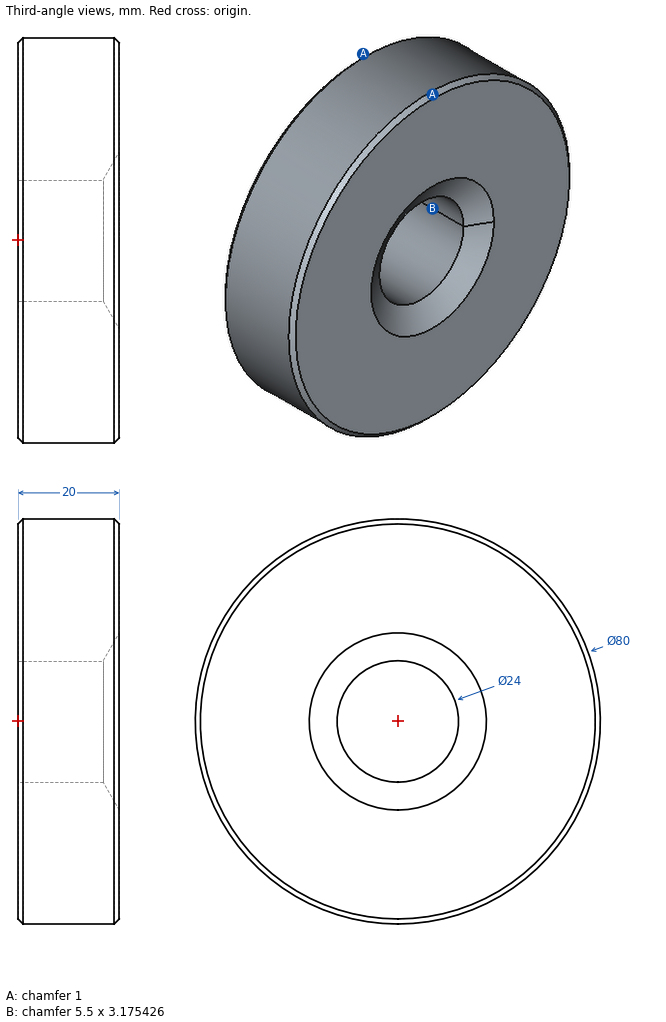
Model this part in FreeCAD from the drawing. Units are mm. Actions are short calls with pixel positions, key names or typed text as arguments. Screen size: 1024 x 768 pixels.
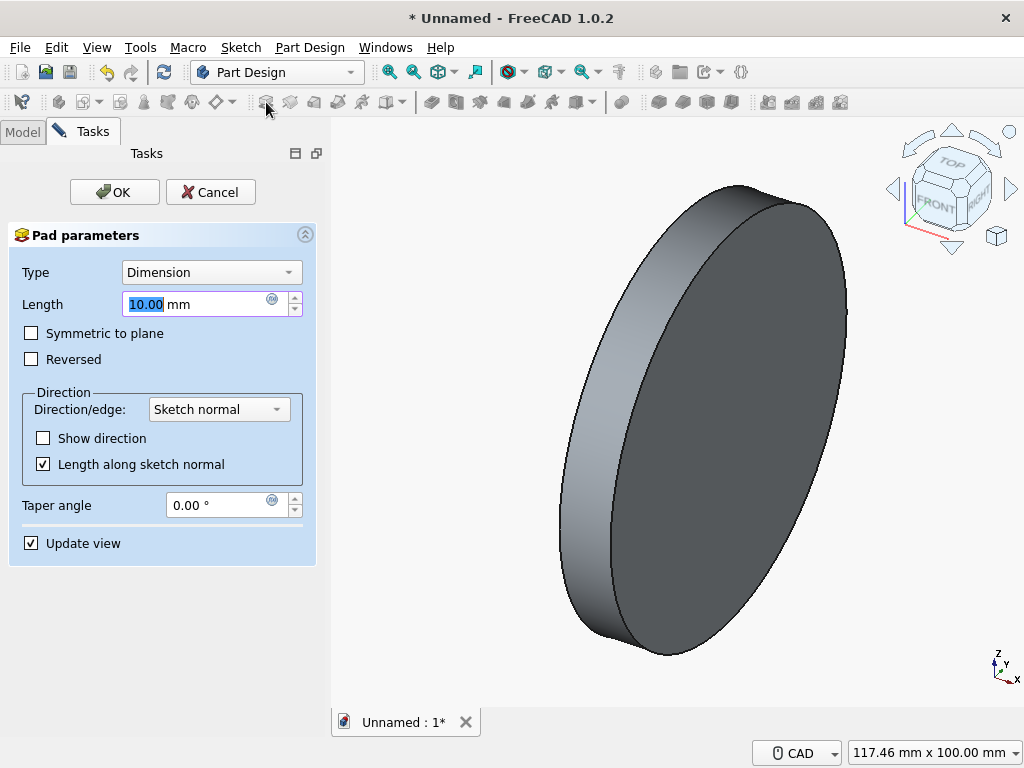
text(20)
key(Tab)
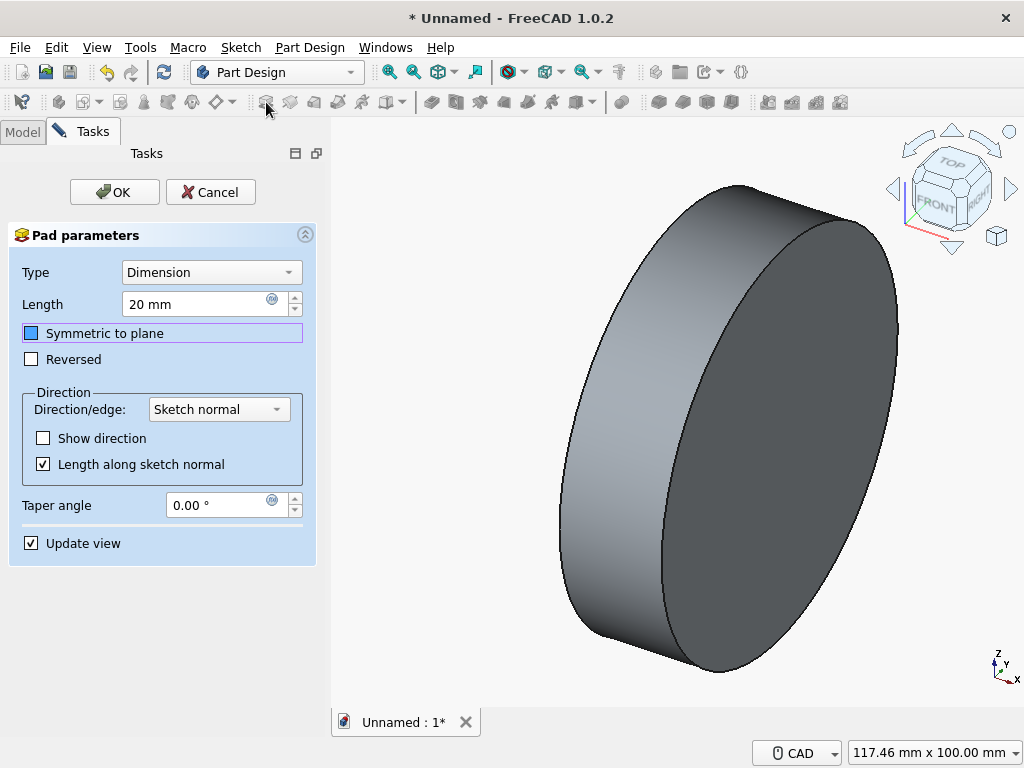
click(115, 192)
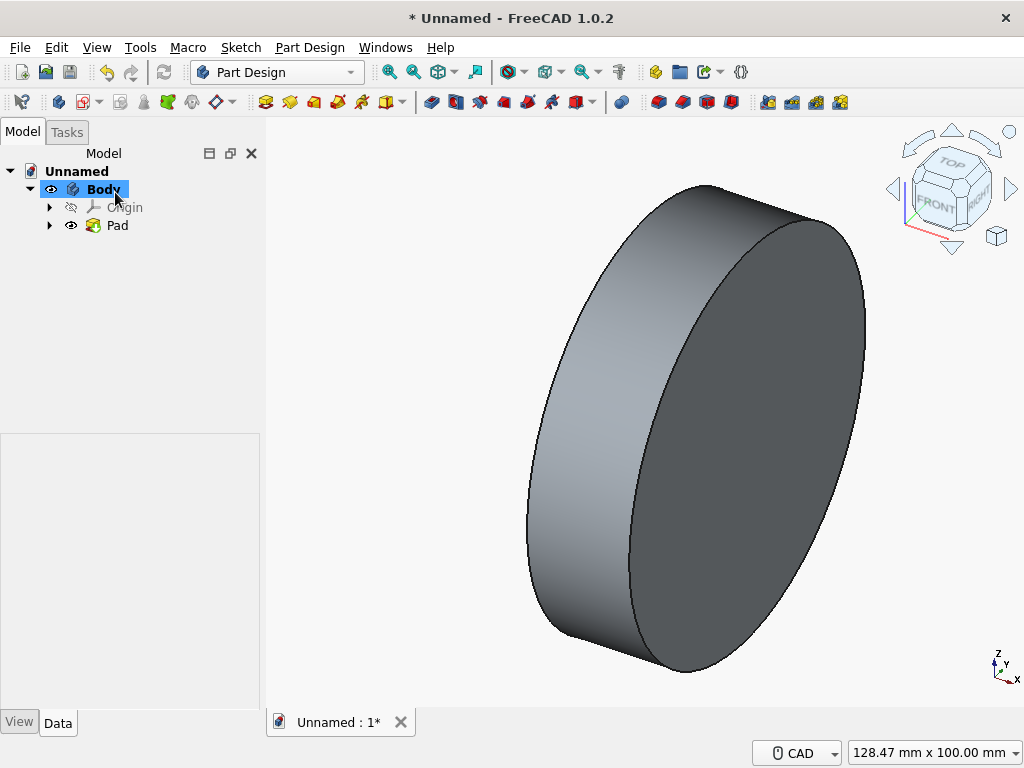
click(390, 72)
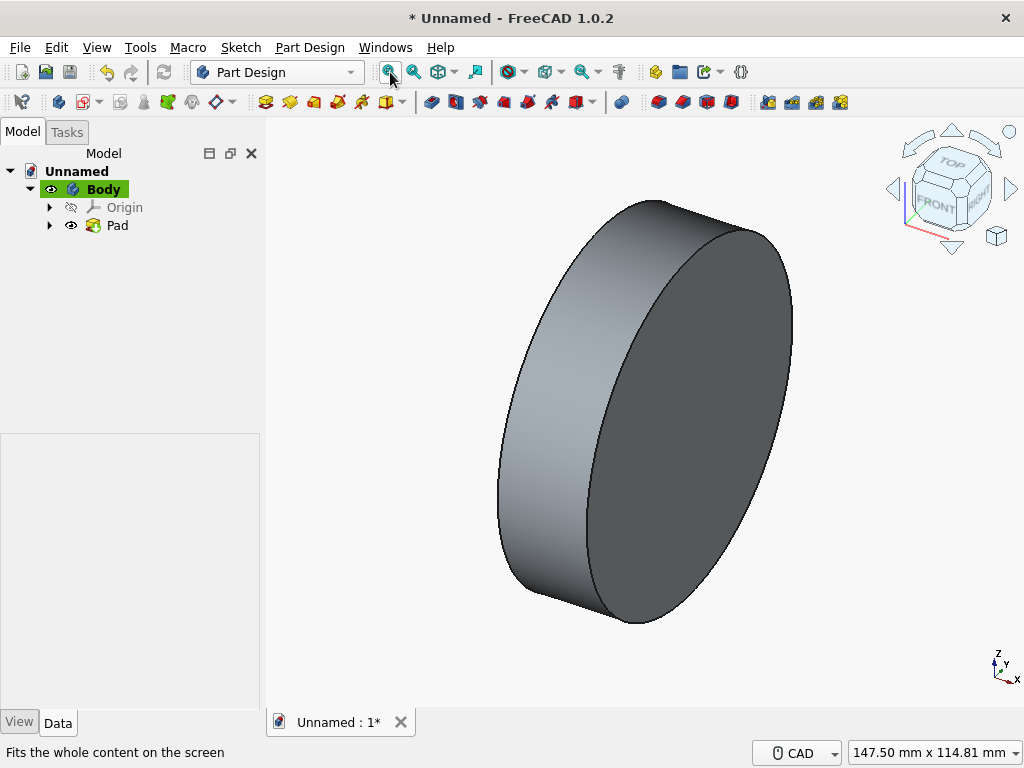
click(690, 426)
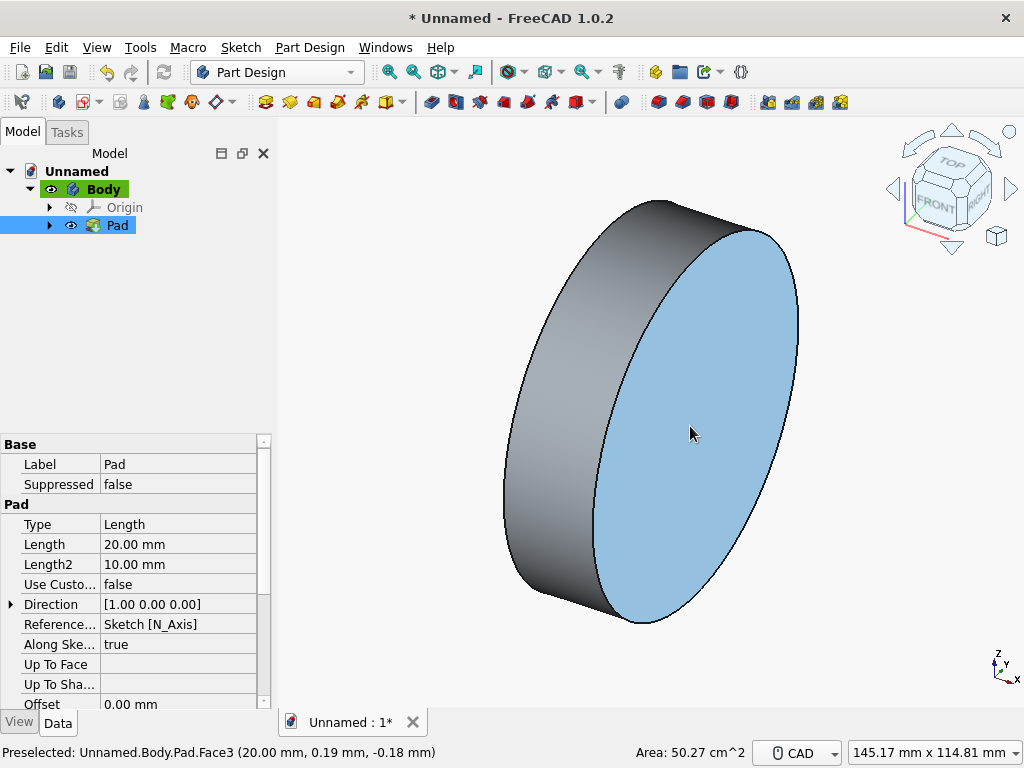
click(84, 102)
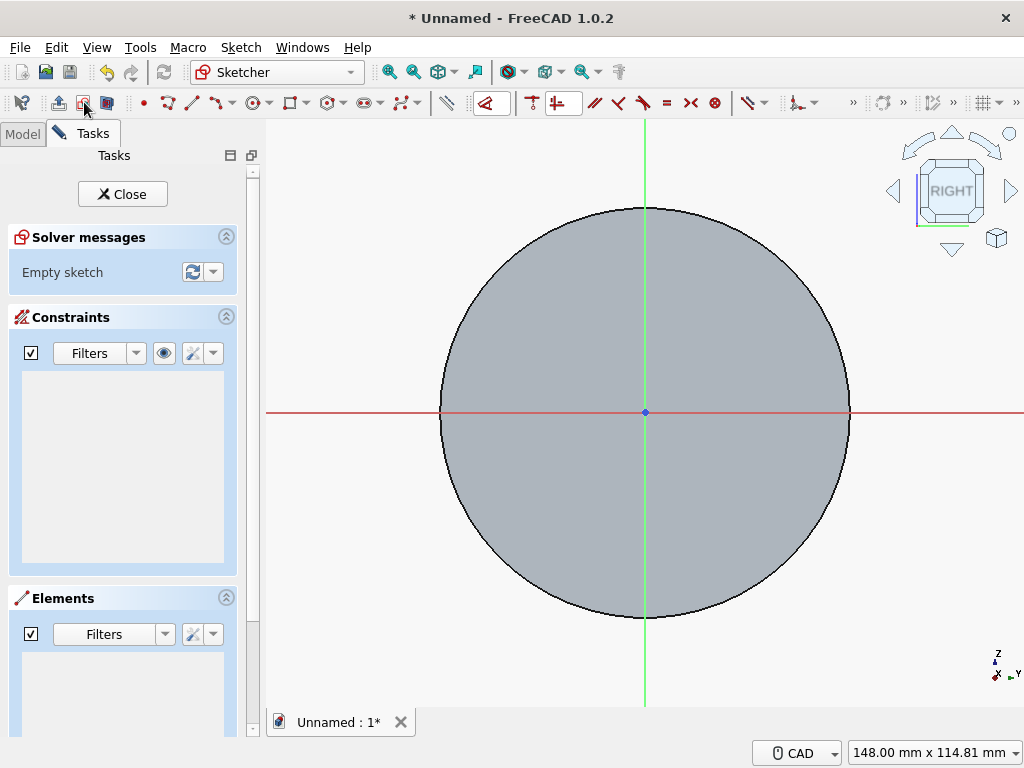
scroll(675, 413, up, 6)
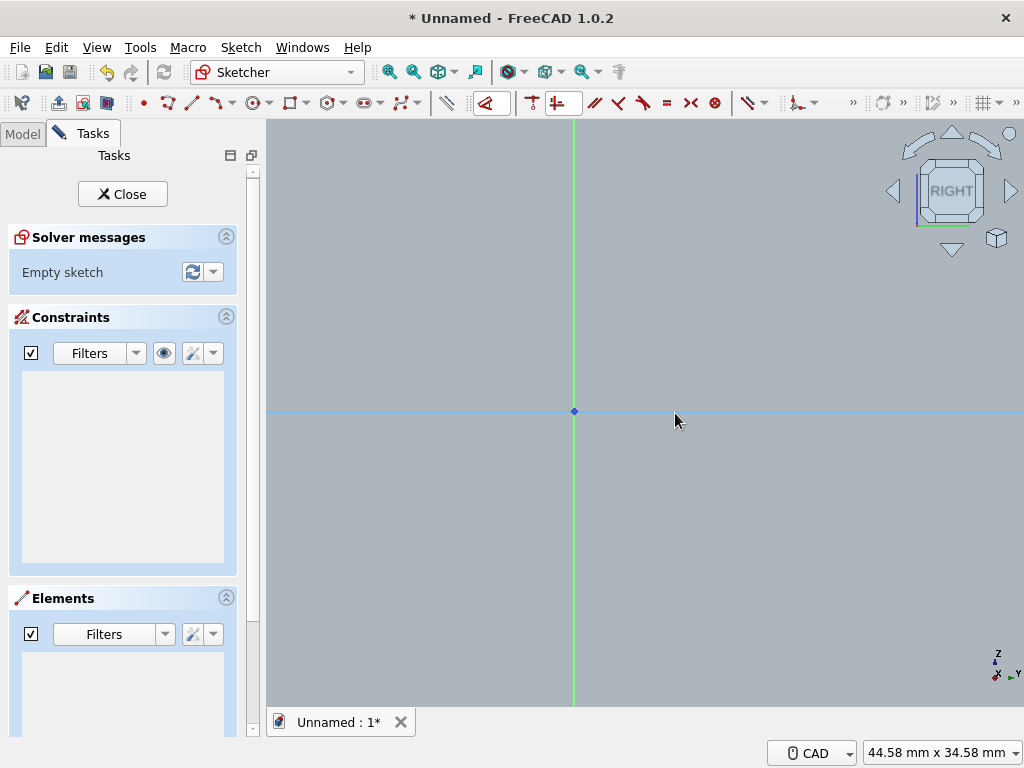
click(254, 104)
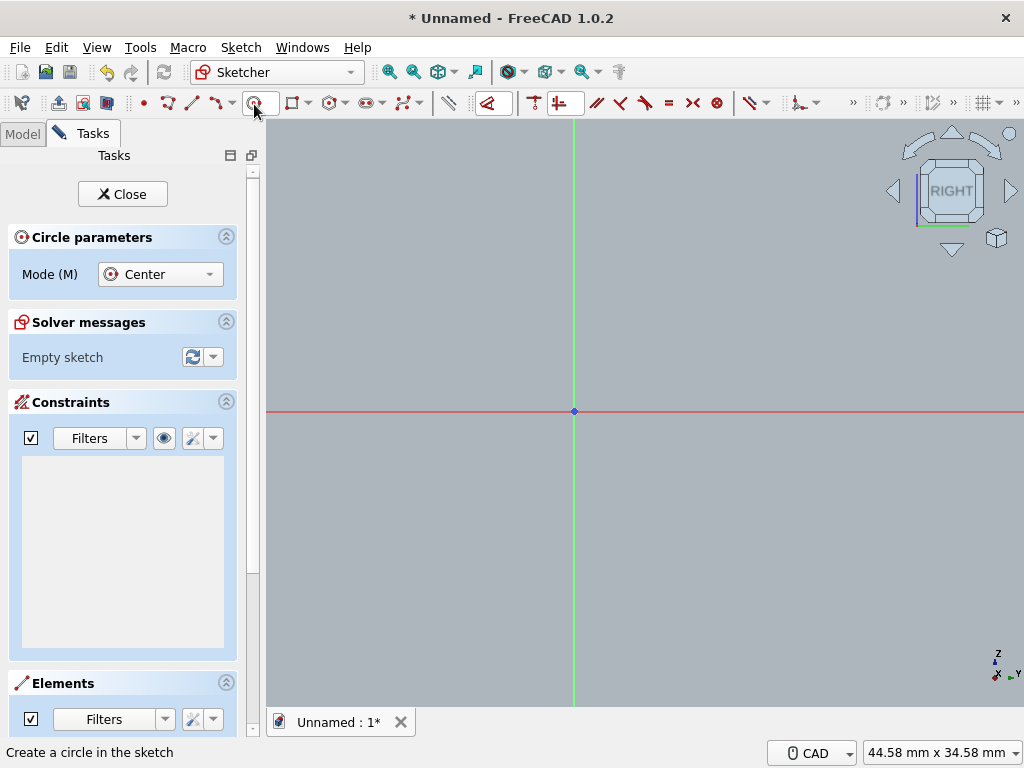
click(574, 412)
click(718, 268)
key(Escape)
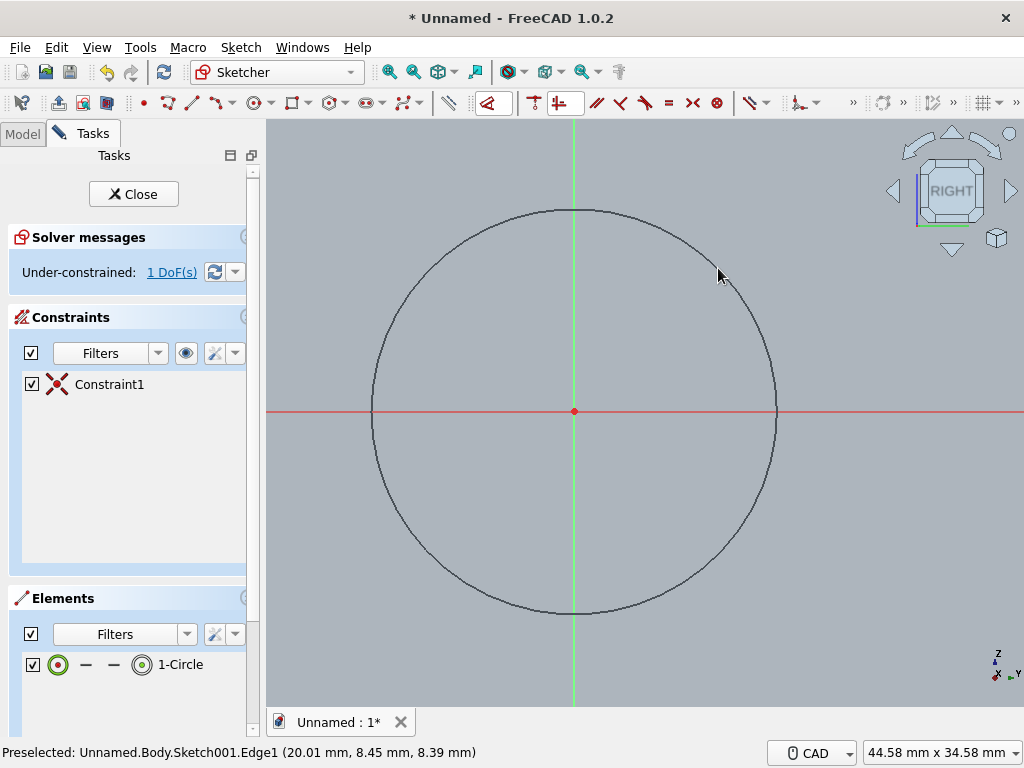
click(717, 268)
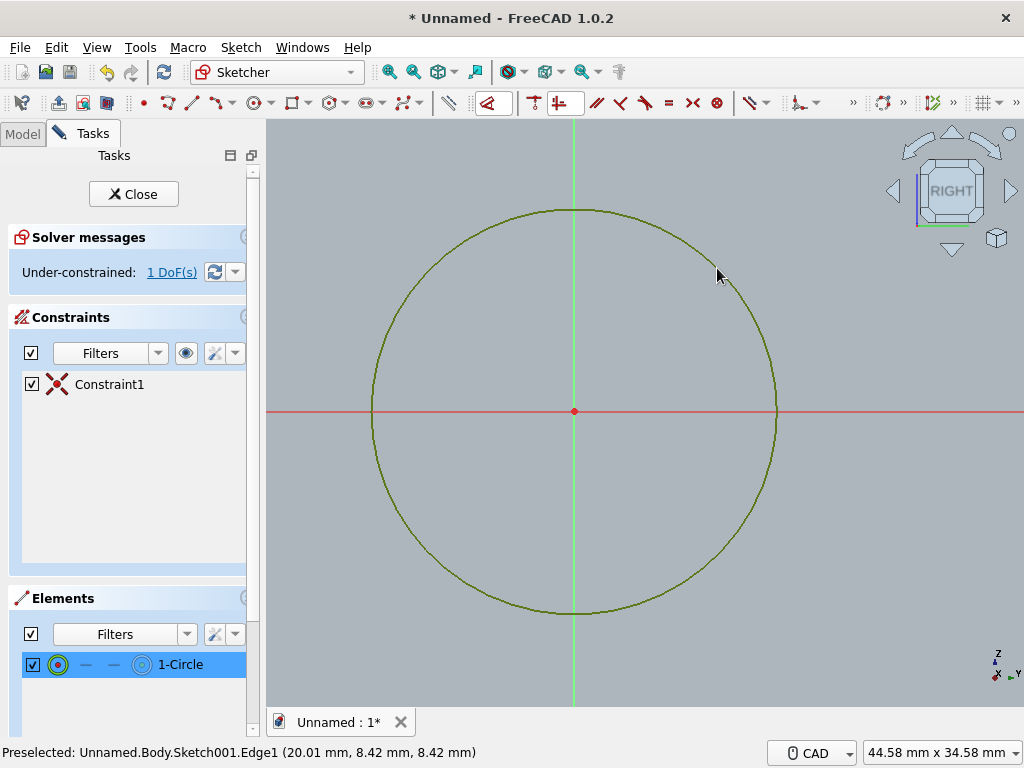
click(506, 104)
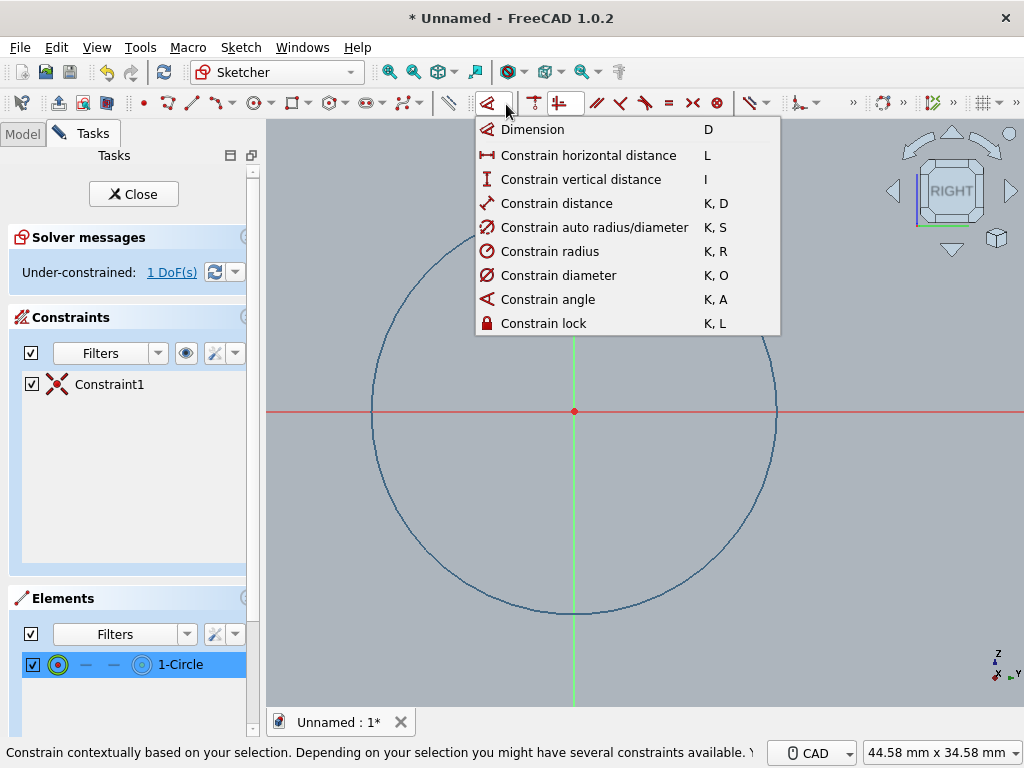
click(628, 275)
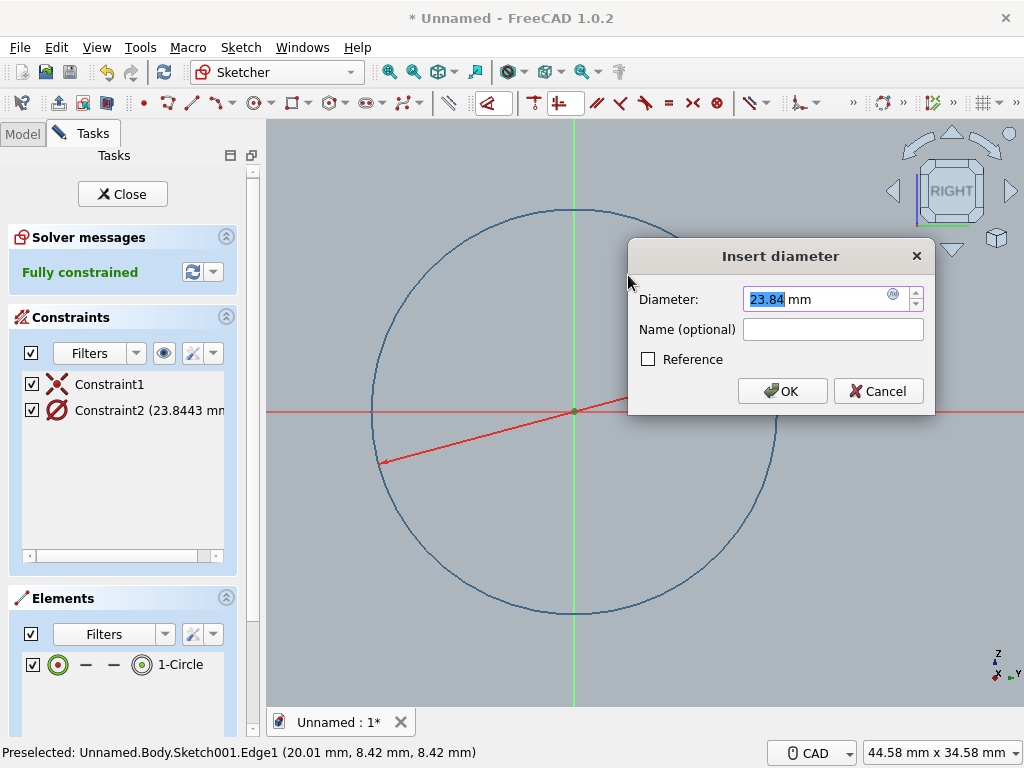
text(24)
key(Return)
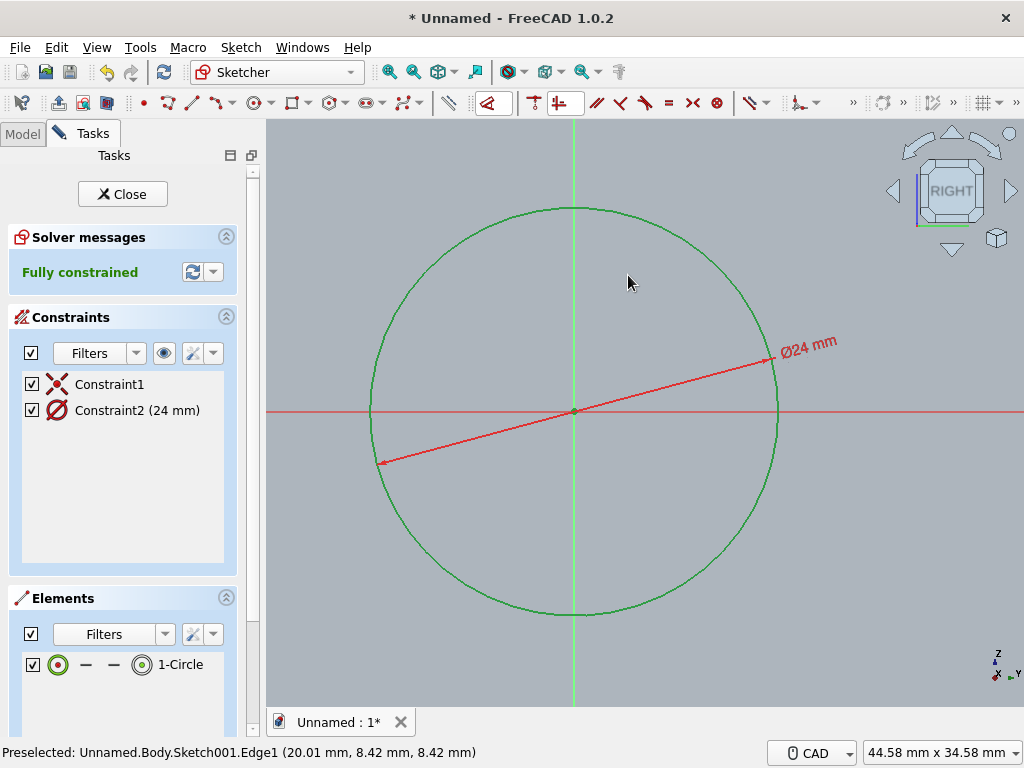
click(123, 194)